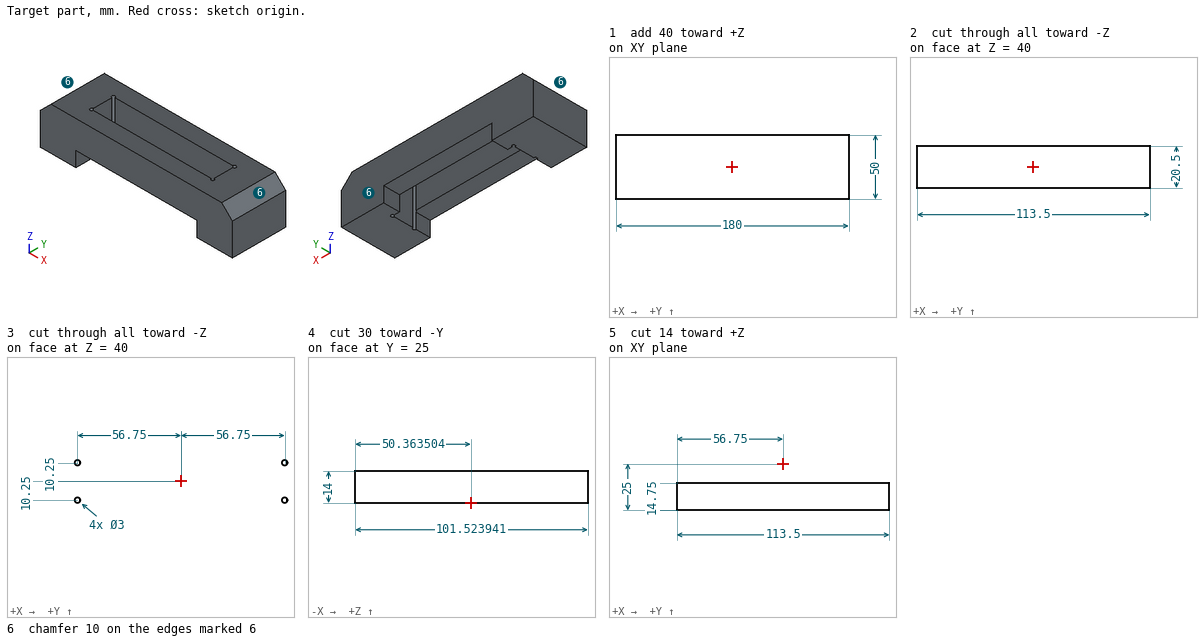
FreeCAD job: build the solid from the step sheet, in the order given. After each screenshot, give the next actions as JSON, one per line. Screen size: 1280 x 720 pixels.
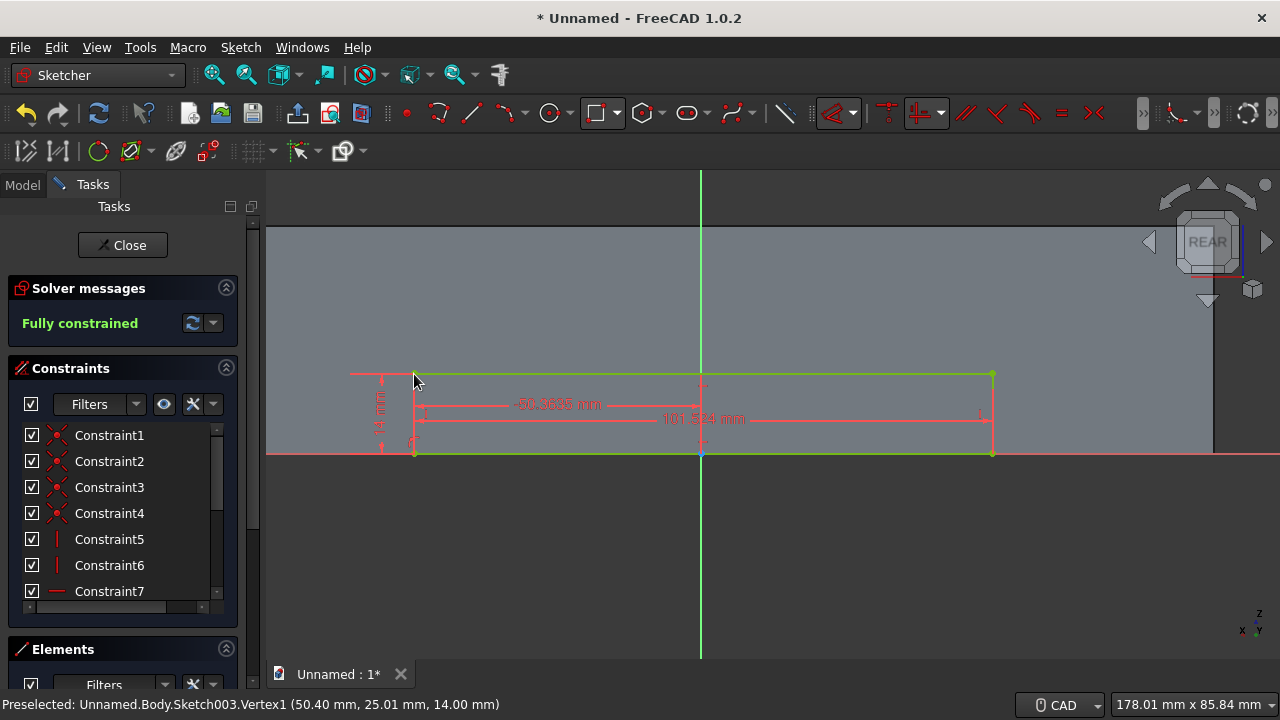
{"action": "left_click", "coordinate": [123, 245]}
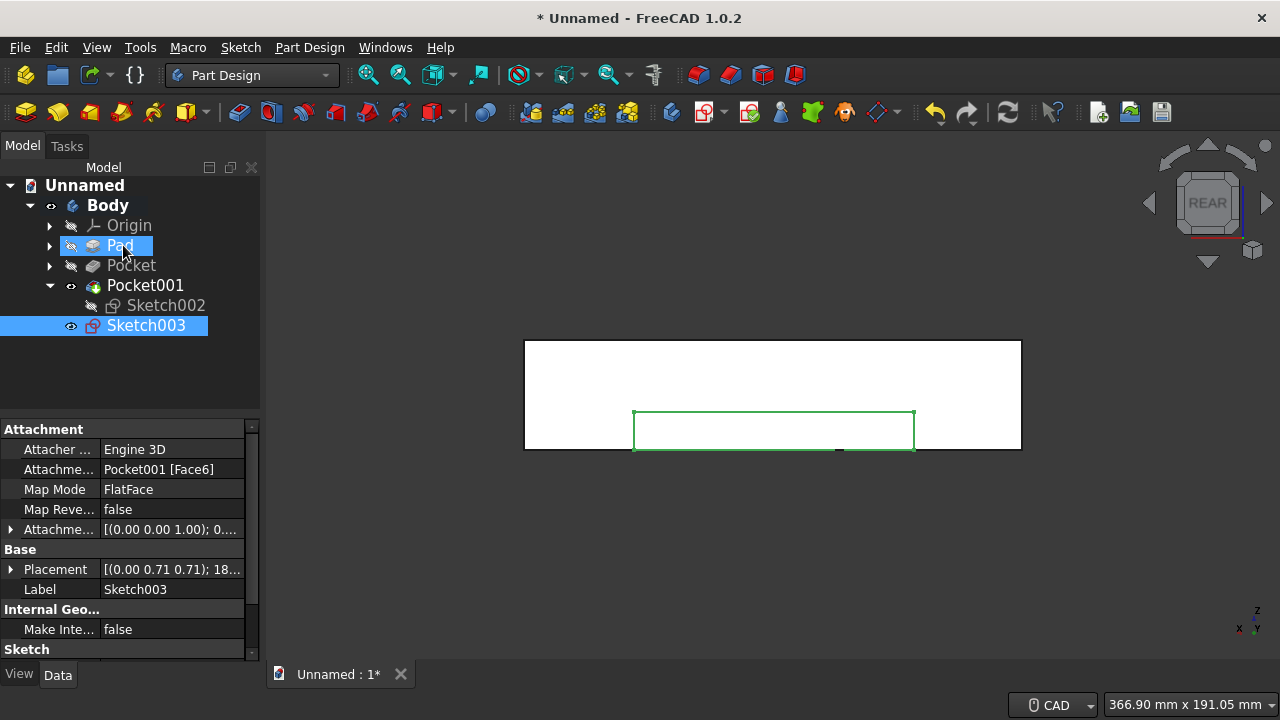
{"action": "left_click", "coordinate": [240, 112]}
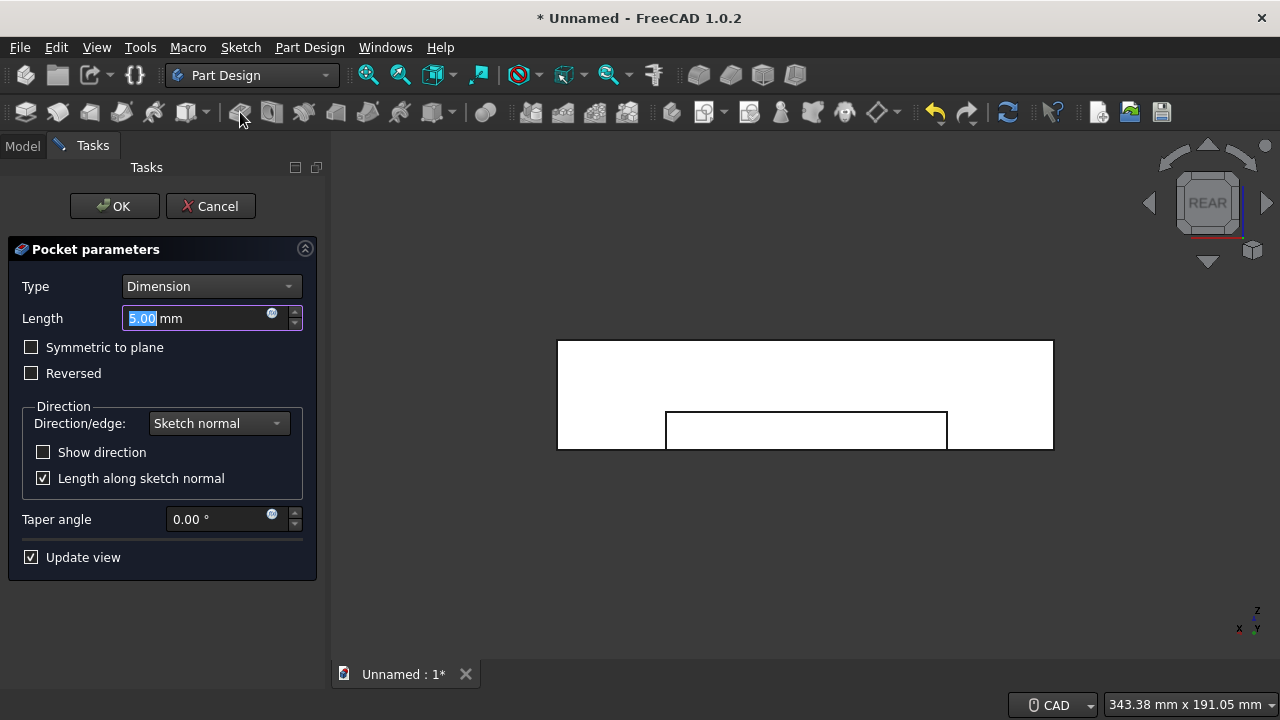
{"action": "type", "text": "30"}
{"action": "key", "text": "Tab"}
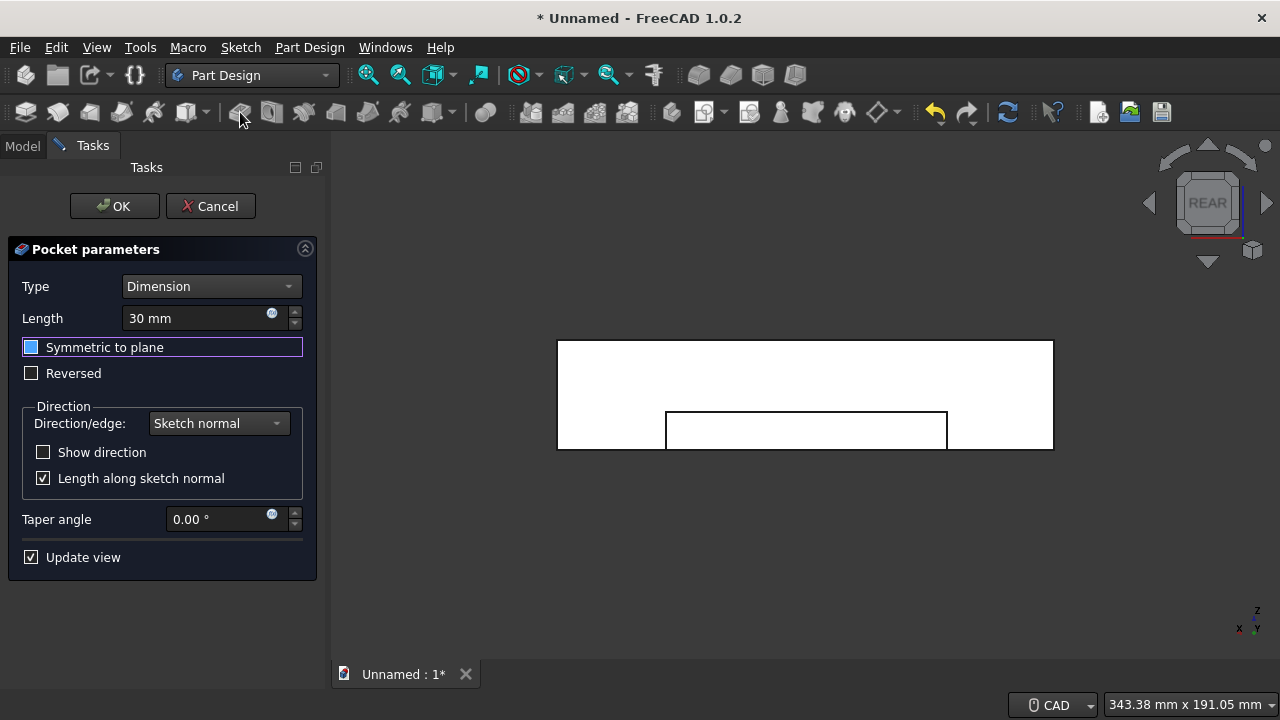
{"action": "left_click", "coordinate": [115, 206]}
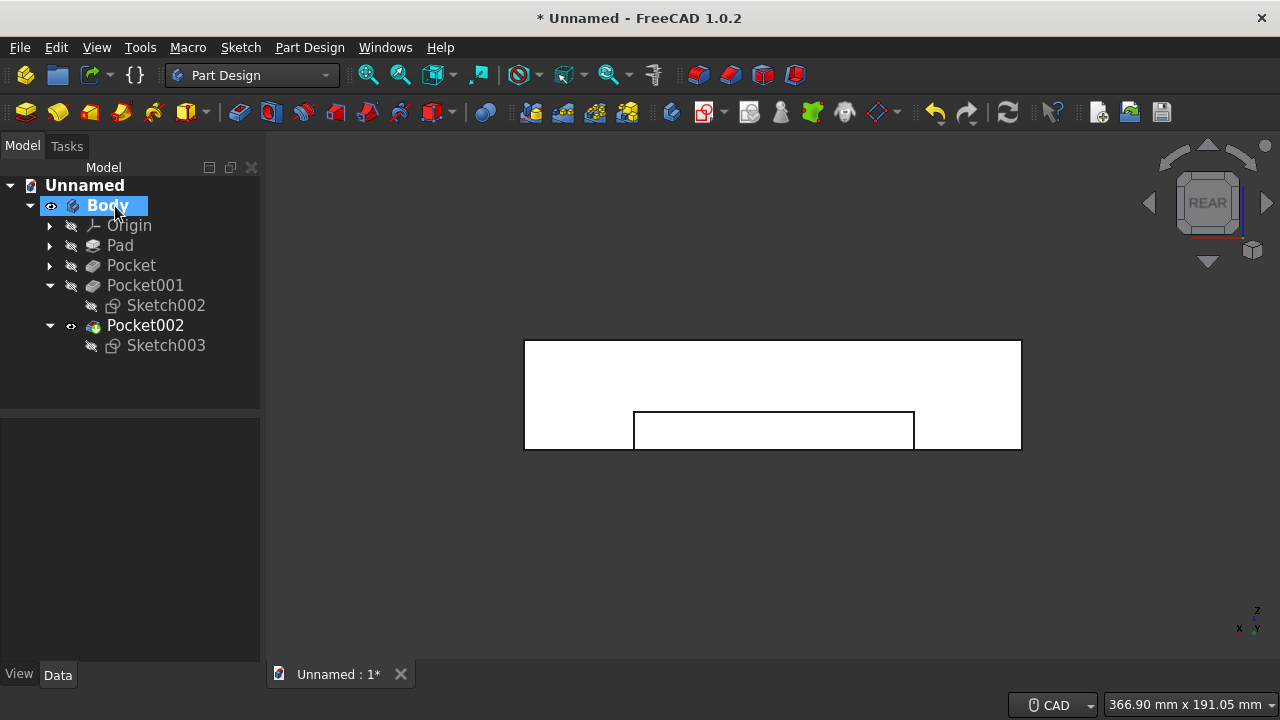
{"action": "left_click", "coordinate": [704, 112]}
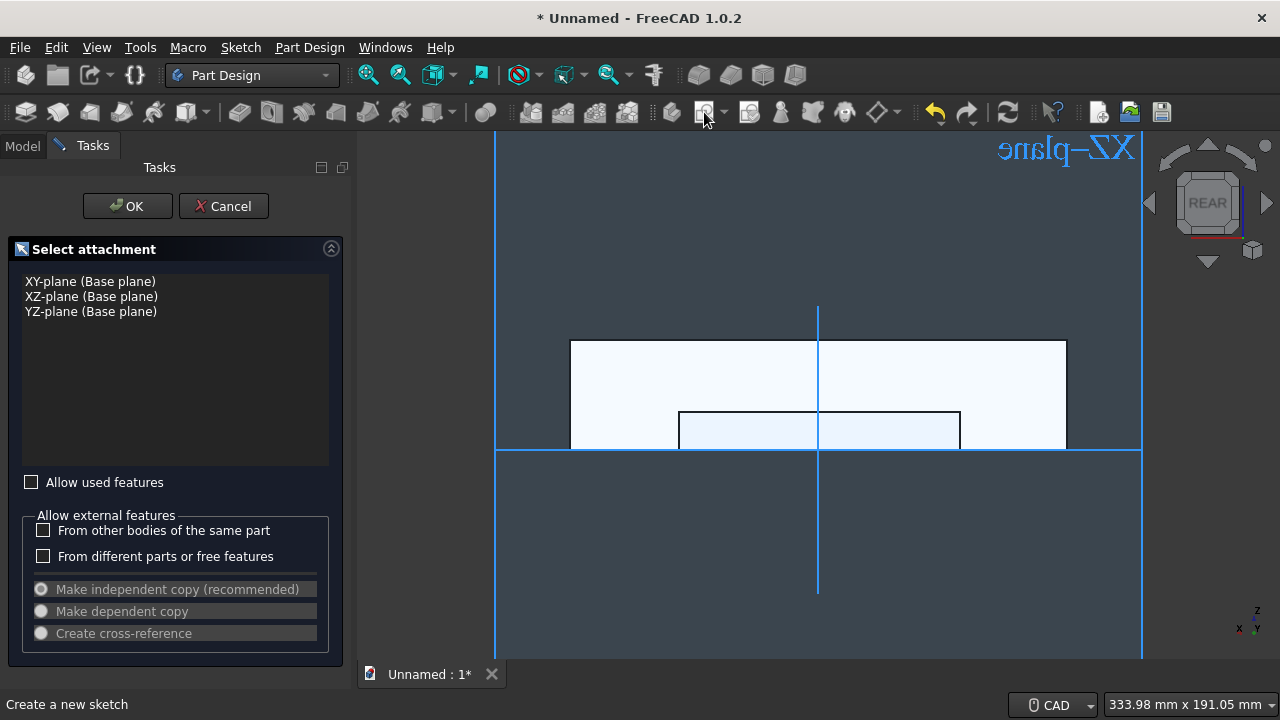
{"action": "left_click", "coordinate": [82, 282]}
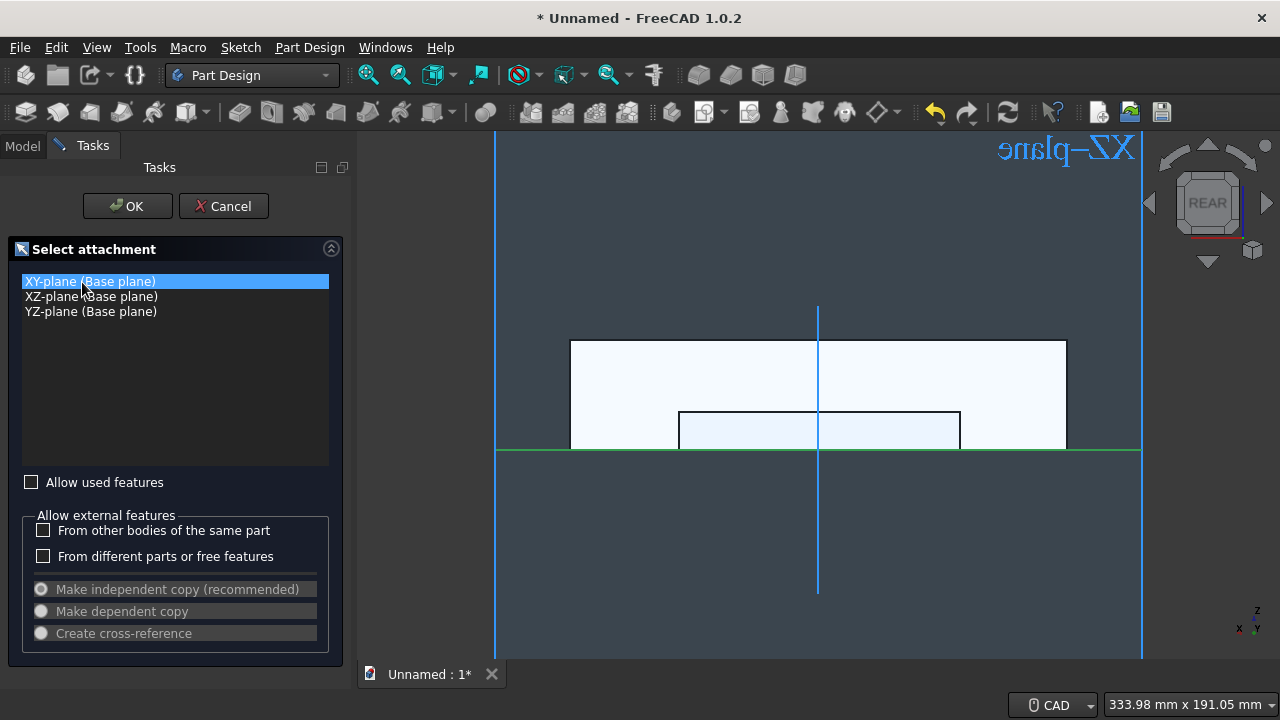
{"action": "left_click", "coordinate": [128, 206]}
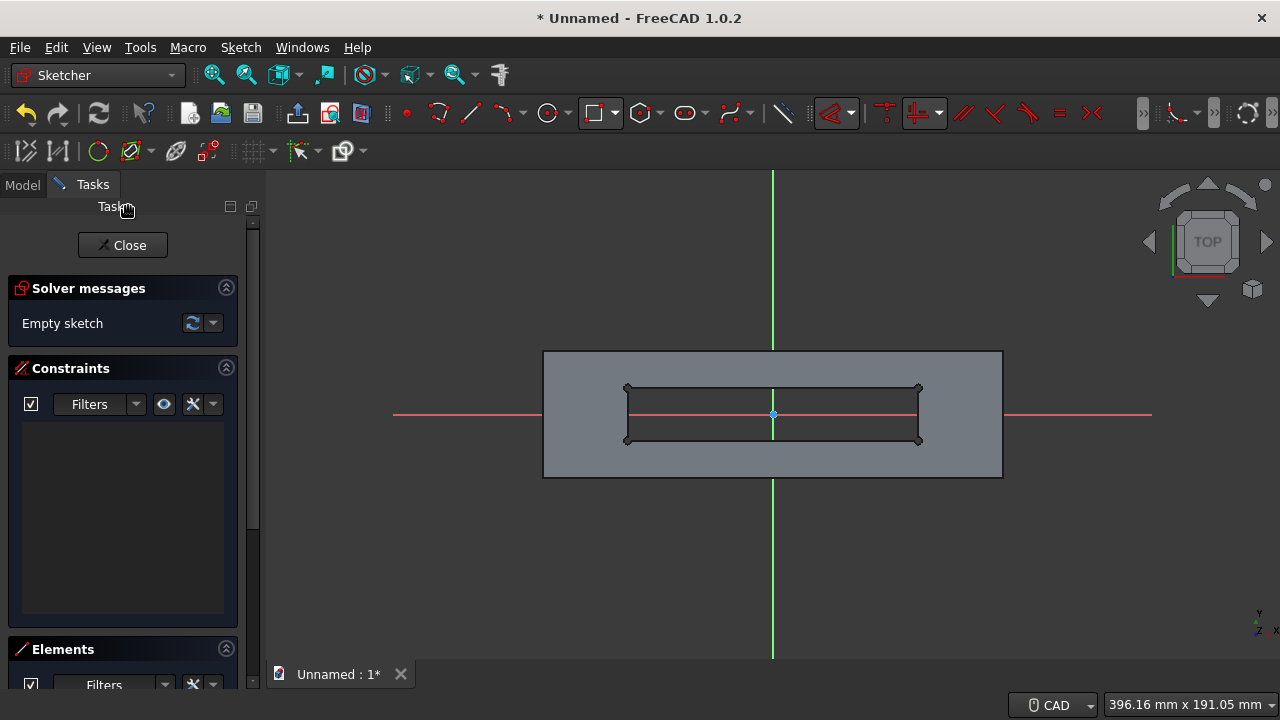
{"action": "left_click", "coordinate": [362, 114]}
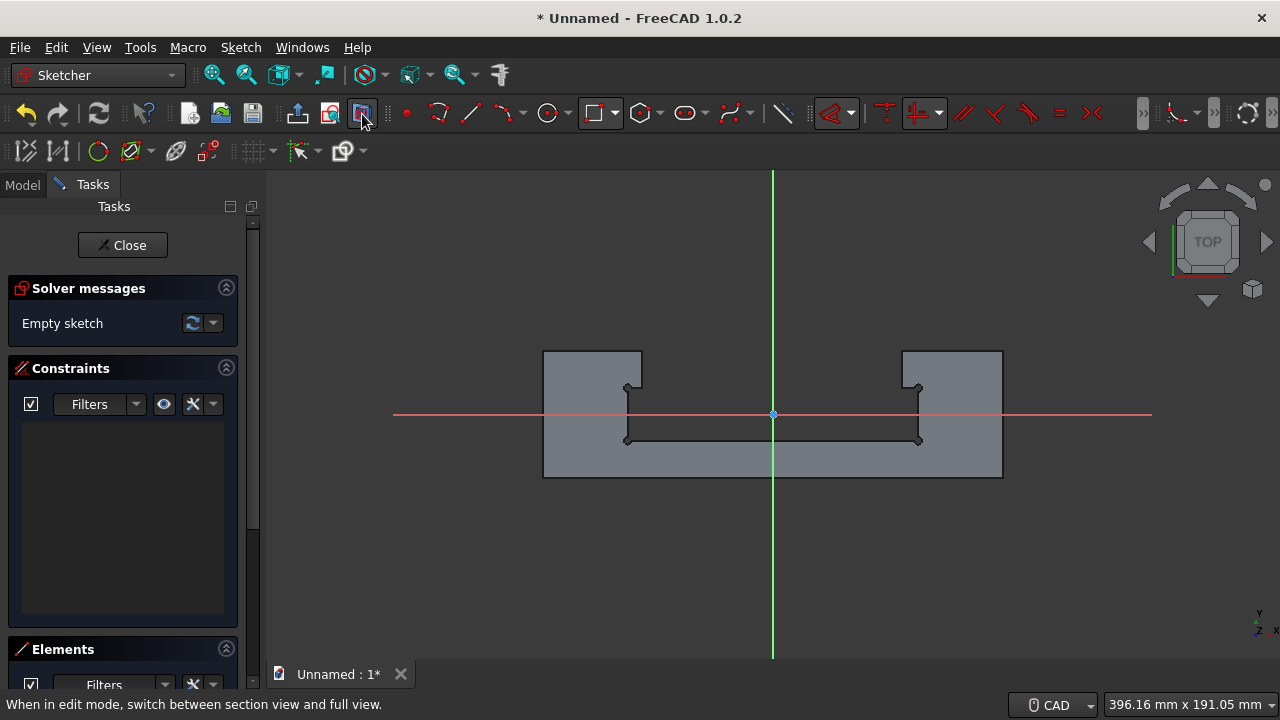
{"action": "scroll", "coordinate": [856, 485], "scroll_direction": "up", "scroll_amount": 3}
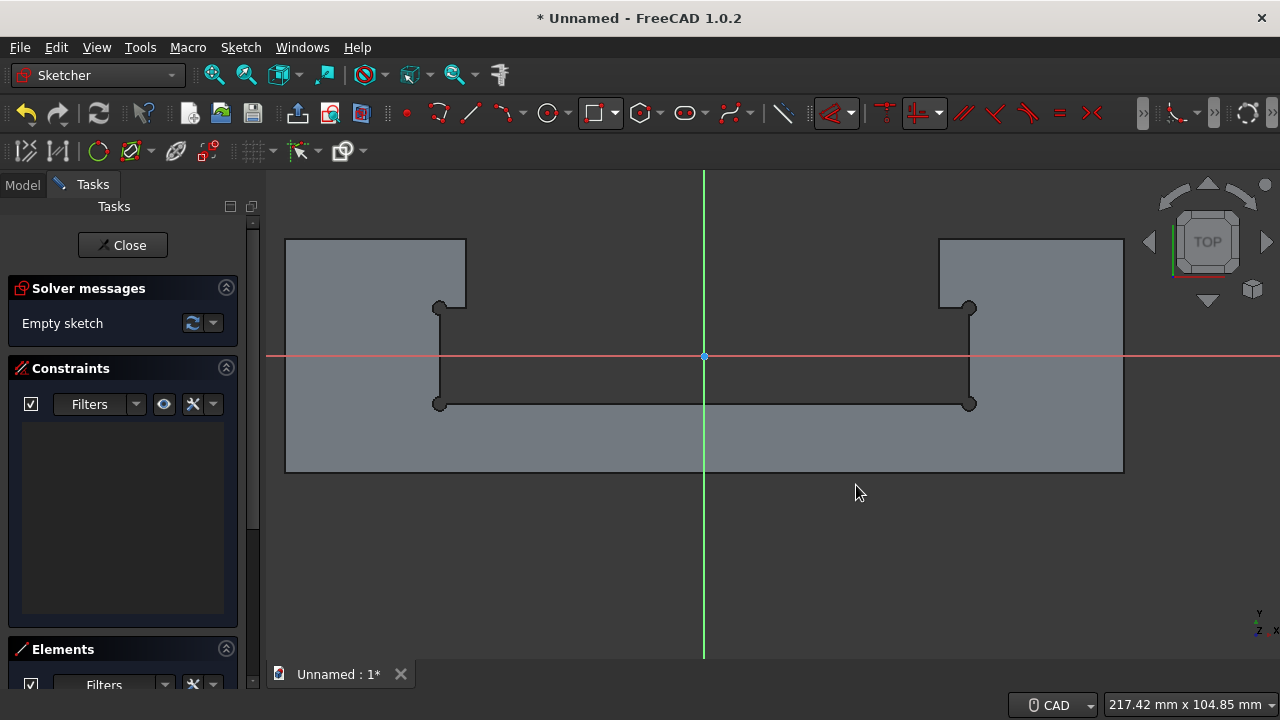
{"action": "left_click", "coordinate": [594, 114]}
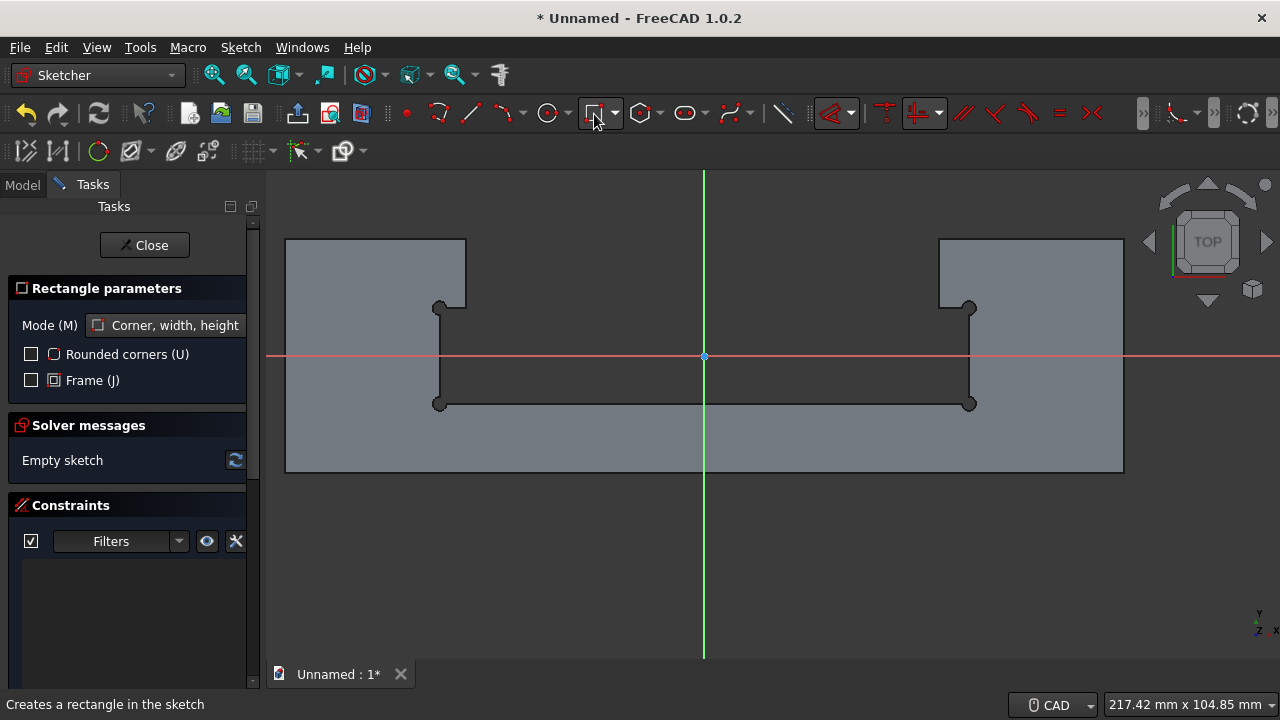
{"action": "left_click", "coordinate": [440, 404]}
{"action": "left_click", "coordinate": [969, 473]}
{"action": "key", "text": "Escape"}